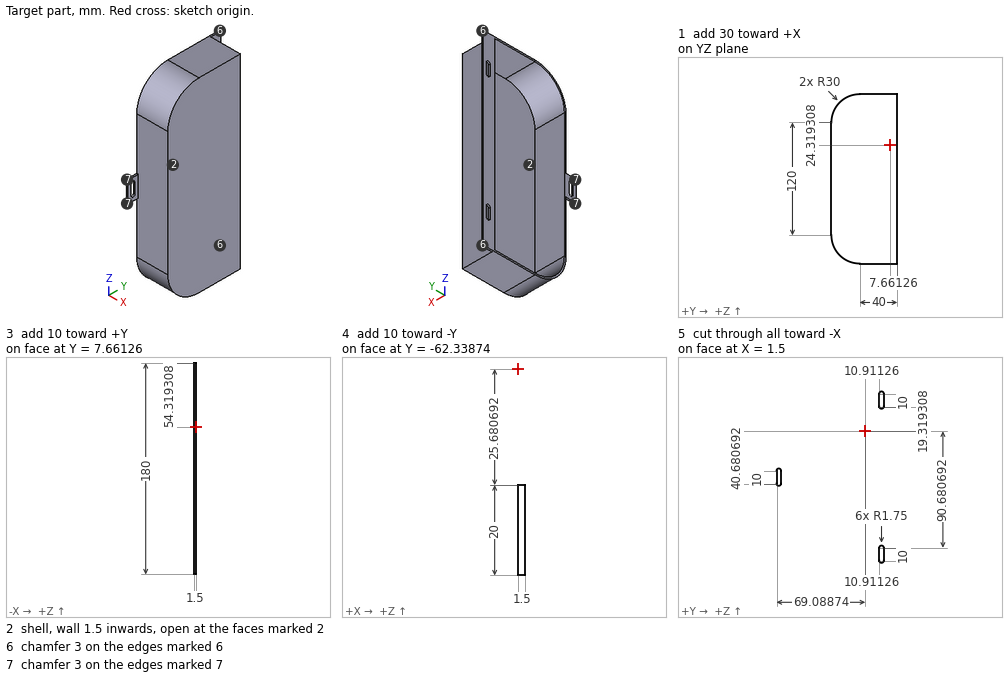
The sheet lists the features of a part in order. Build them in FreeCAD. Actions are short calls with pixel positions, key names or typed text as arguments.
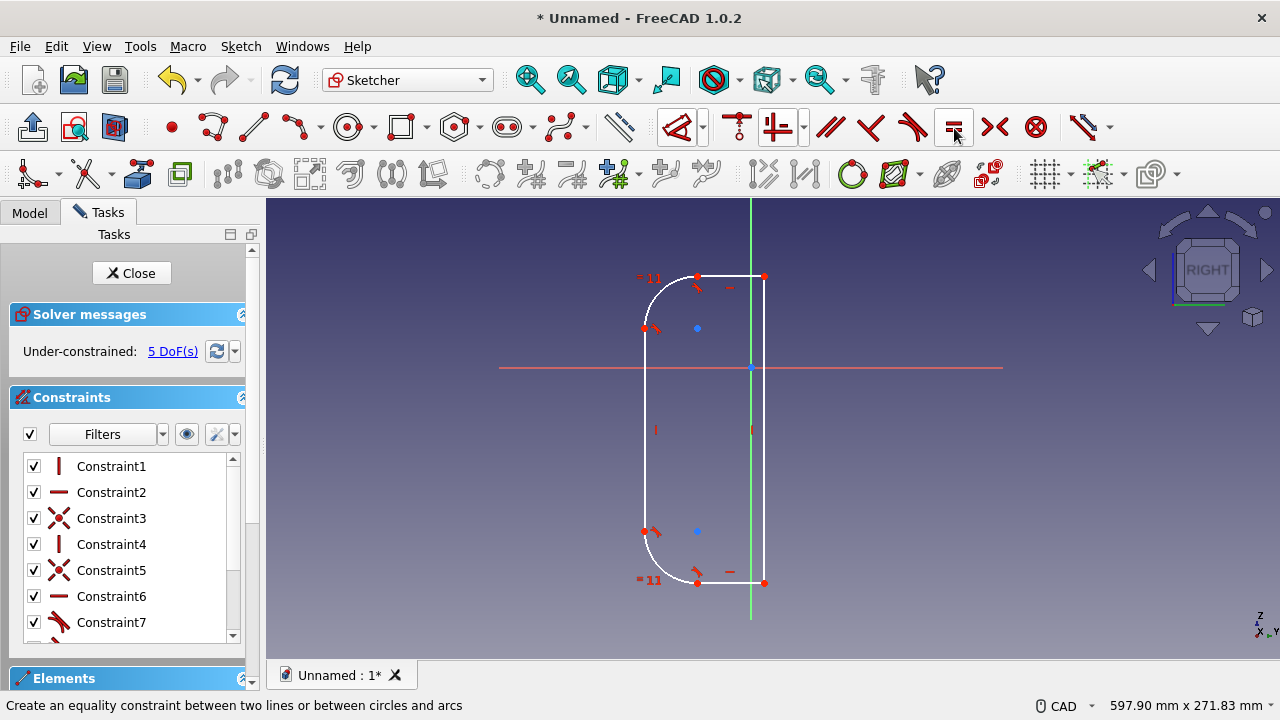
click(676, 128)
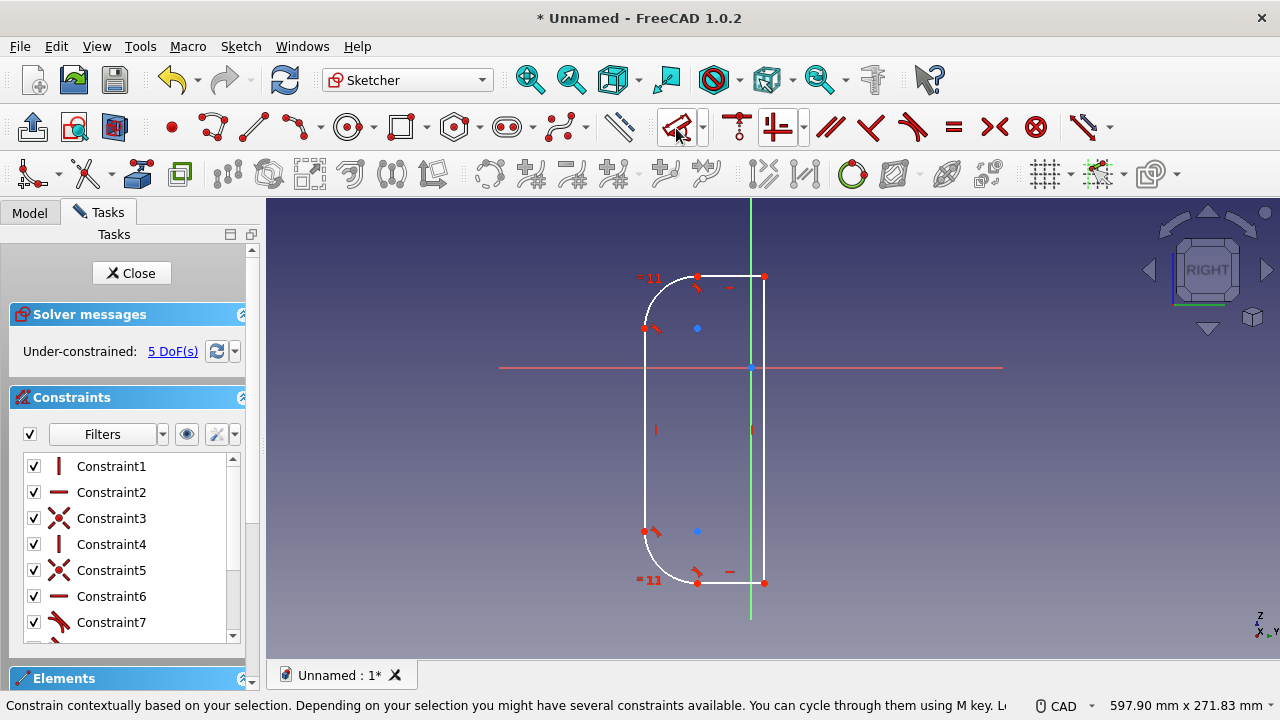
click(651, 555)
click(623, 570)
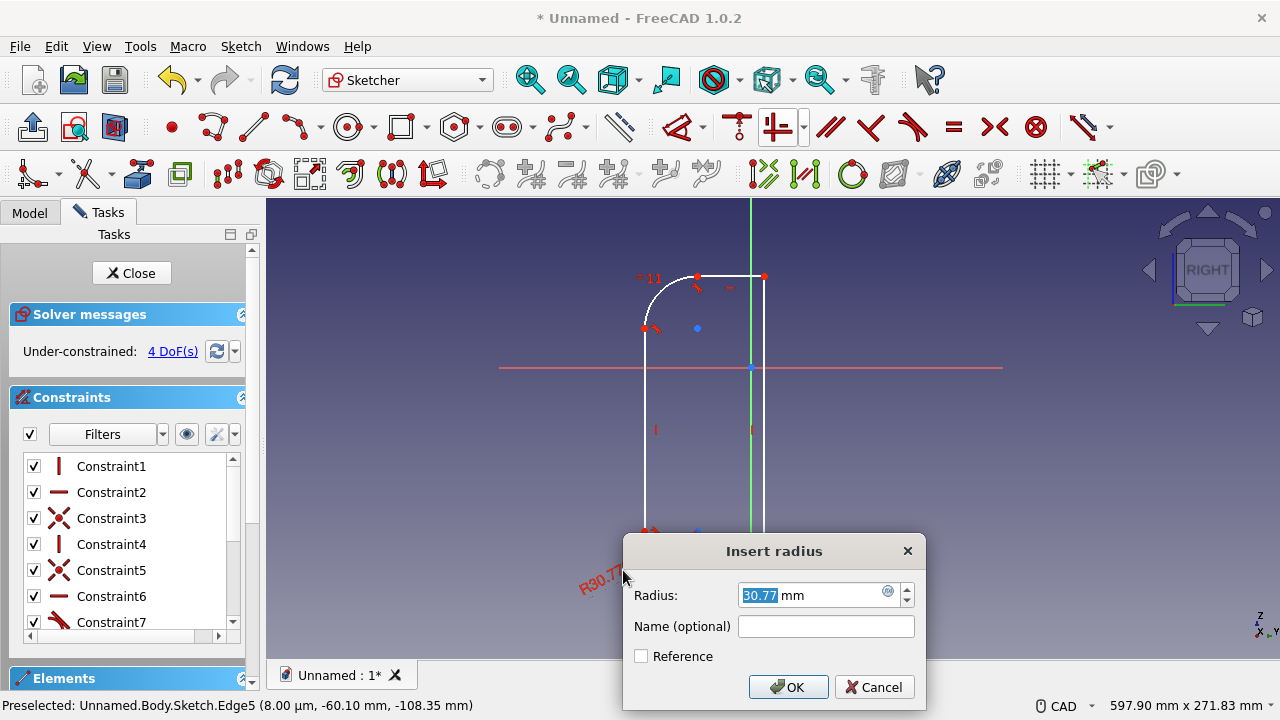
text(30)
key(Return)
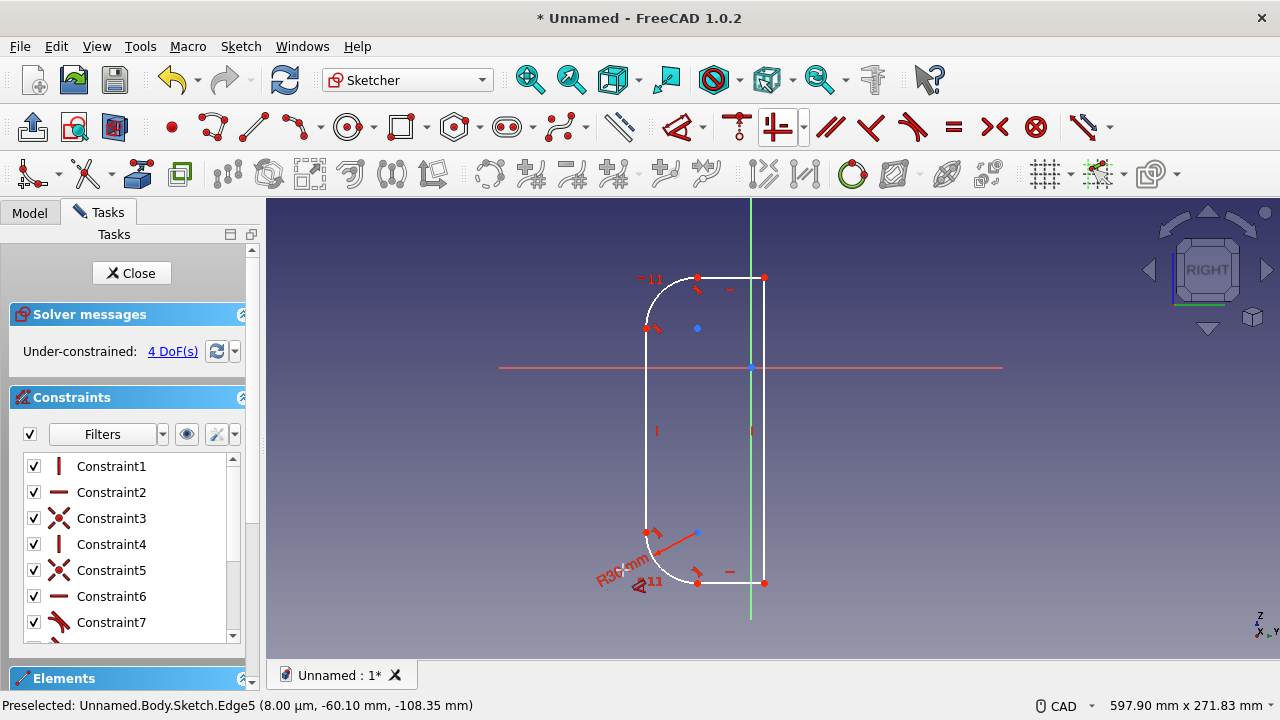
click(717, 583)
click(731, 617)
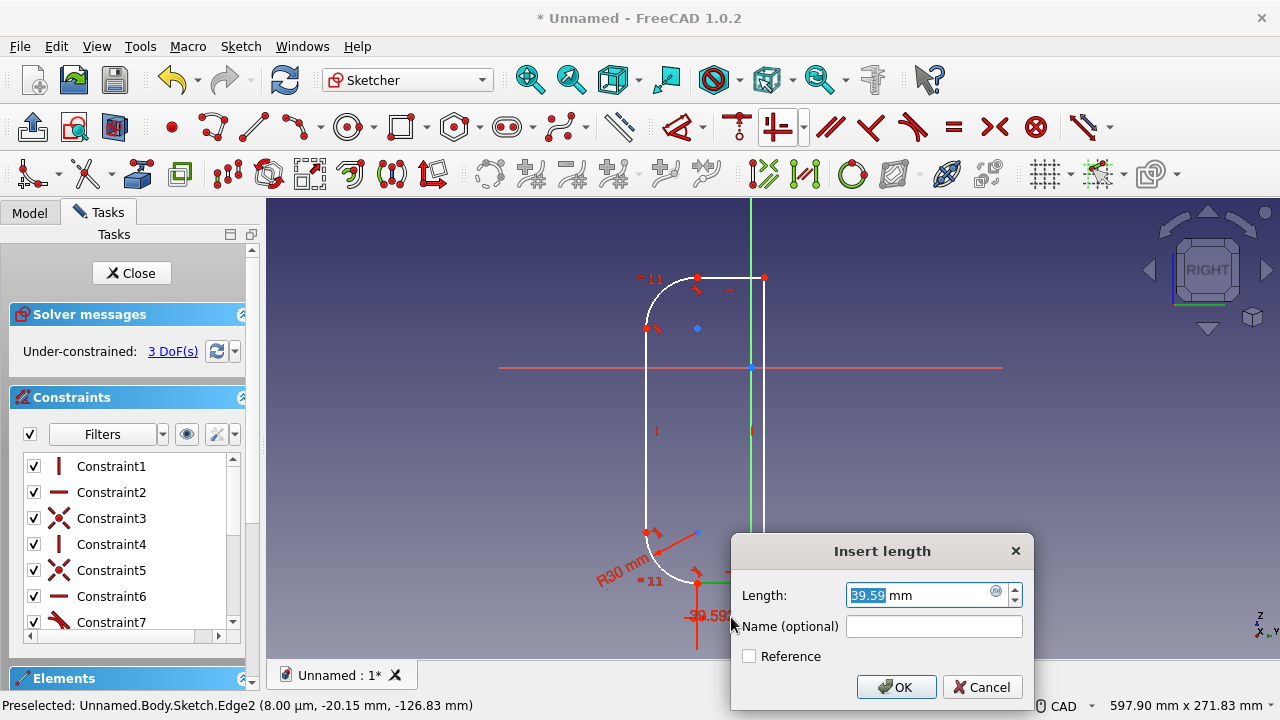
text(40)
key(Return)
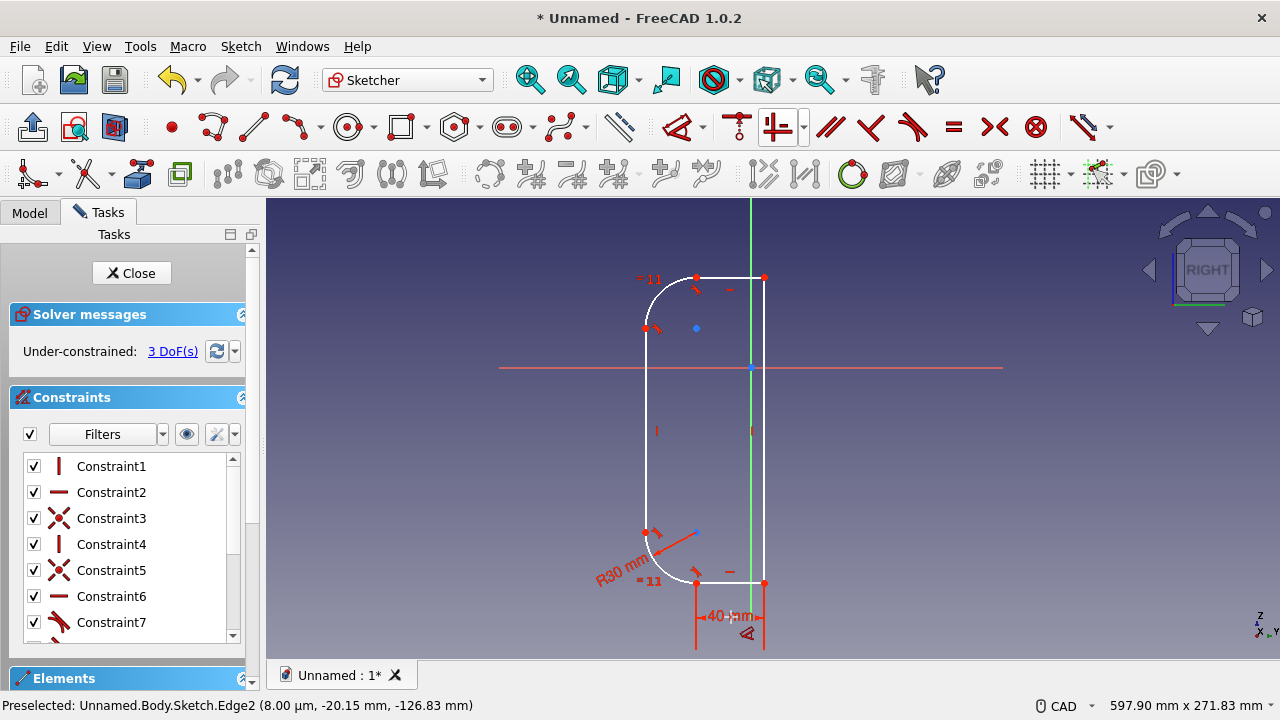
click(646, 390)
click(612, 430)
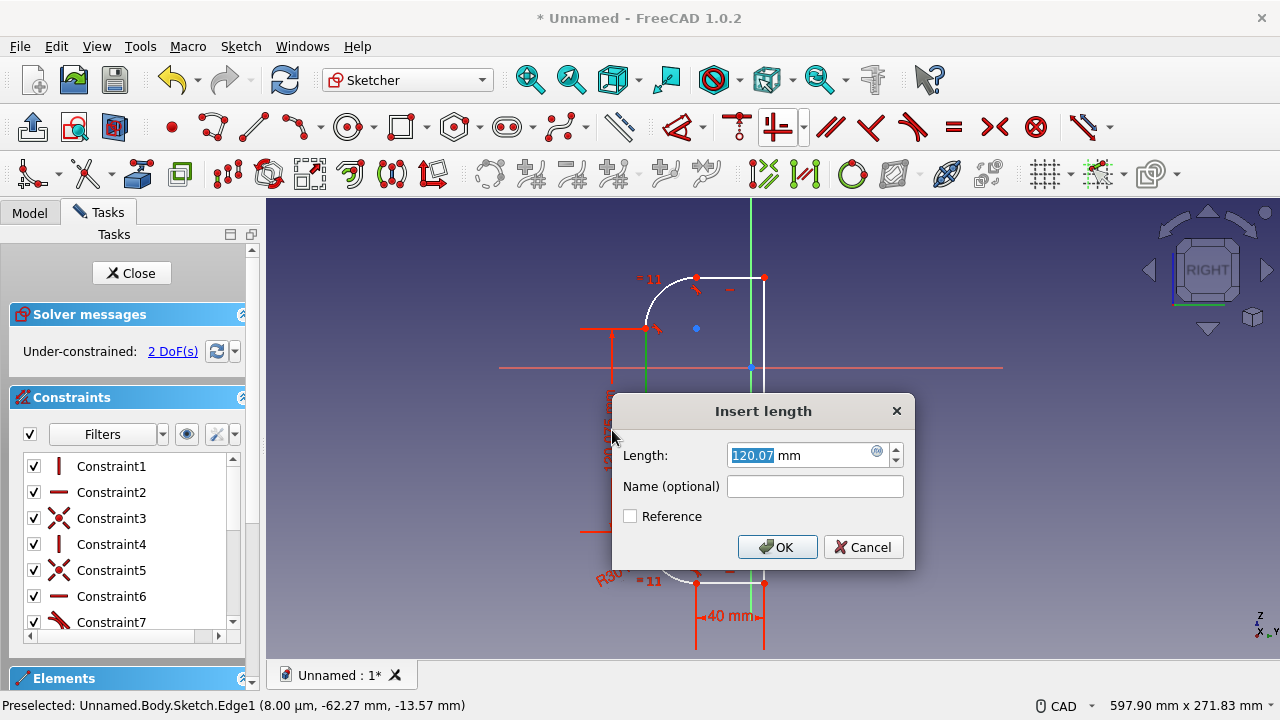
text(120)
key(Return)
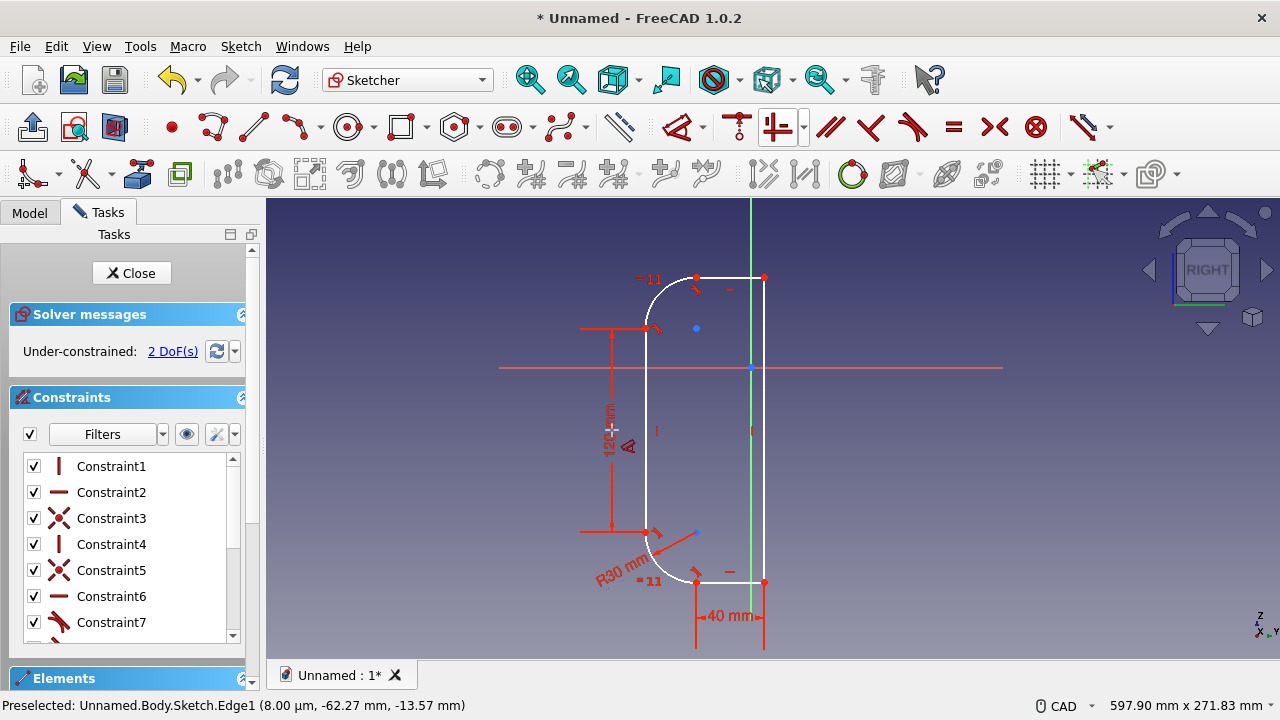
scroll(764, 583, up, 6)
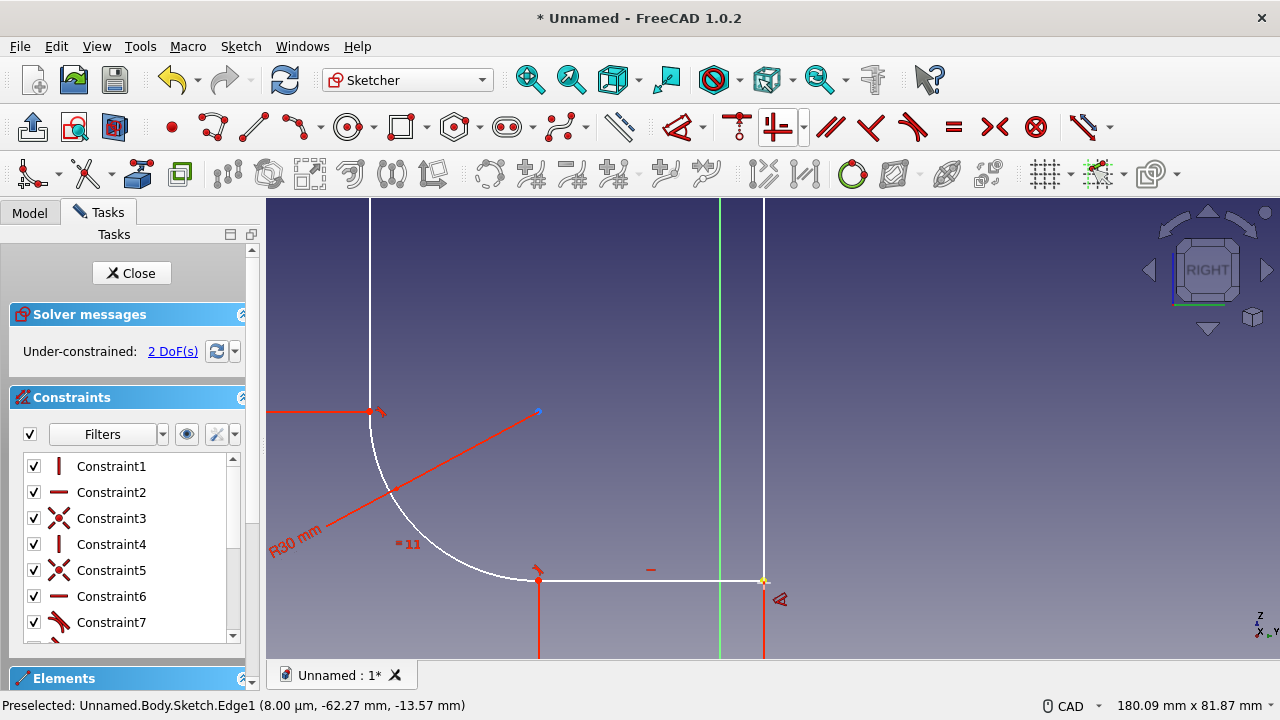
click(764, 581)
click(742, 615)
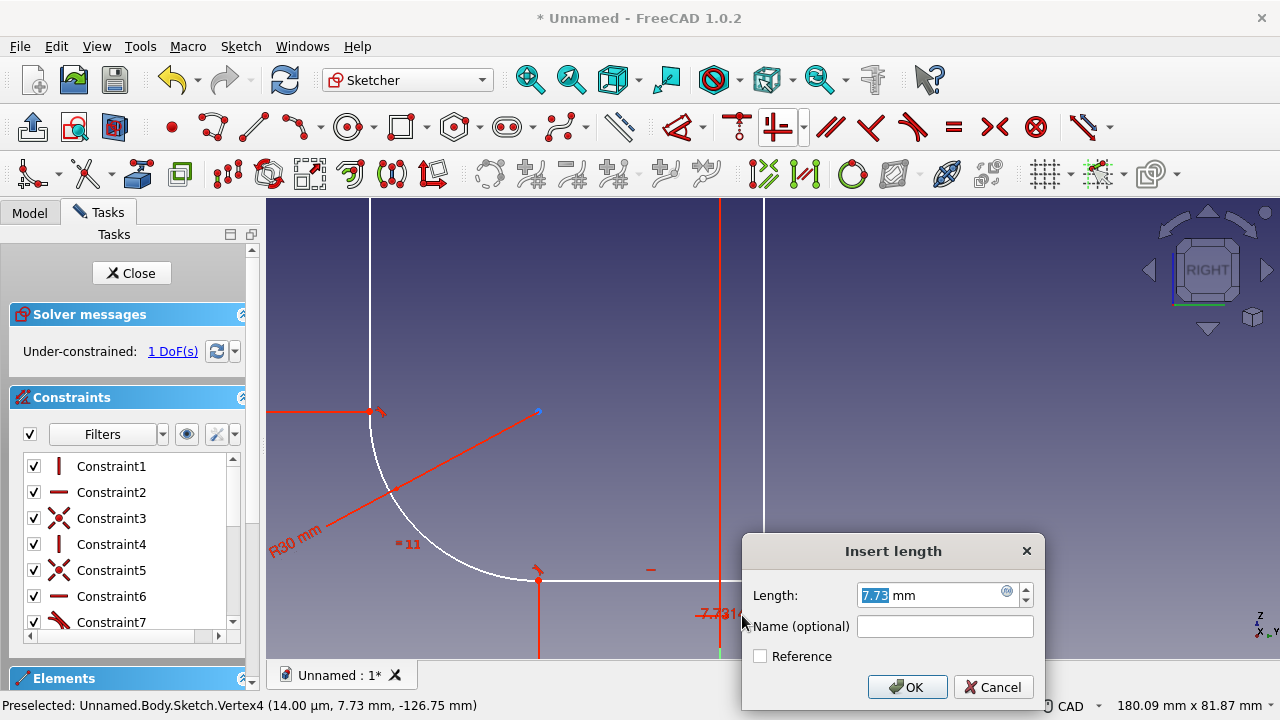
text(7.66126)
key(Return)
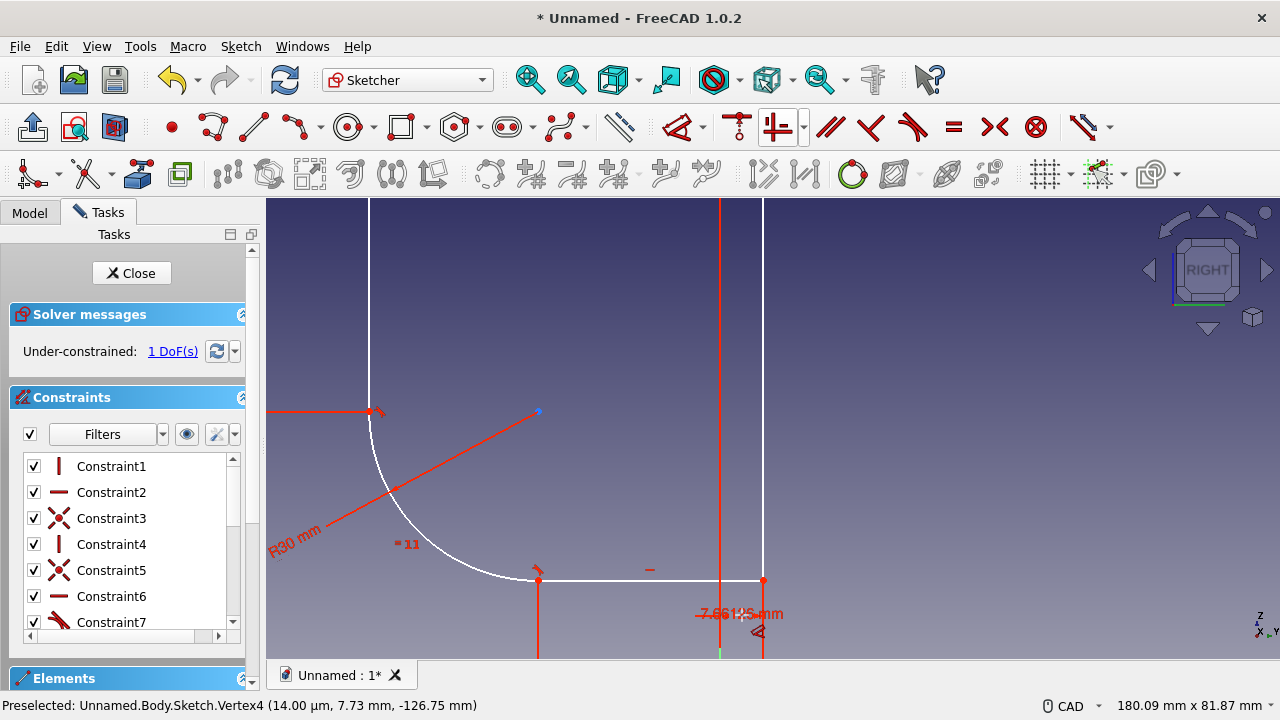
scroll(764, 584, down, 6)